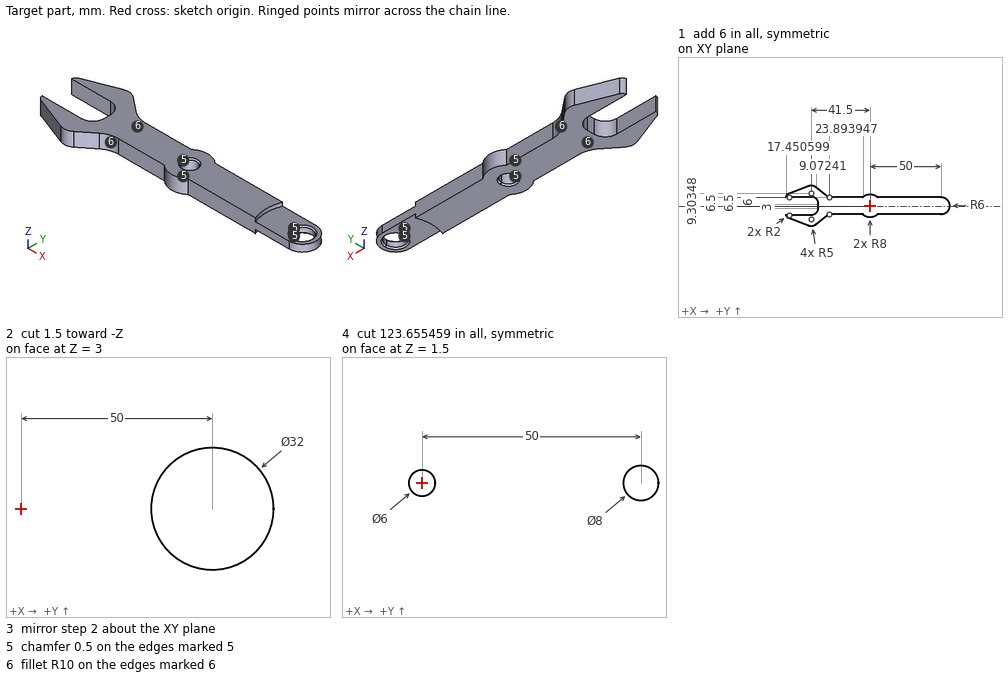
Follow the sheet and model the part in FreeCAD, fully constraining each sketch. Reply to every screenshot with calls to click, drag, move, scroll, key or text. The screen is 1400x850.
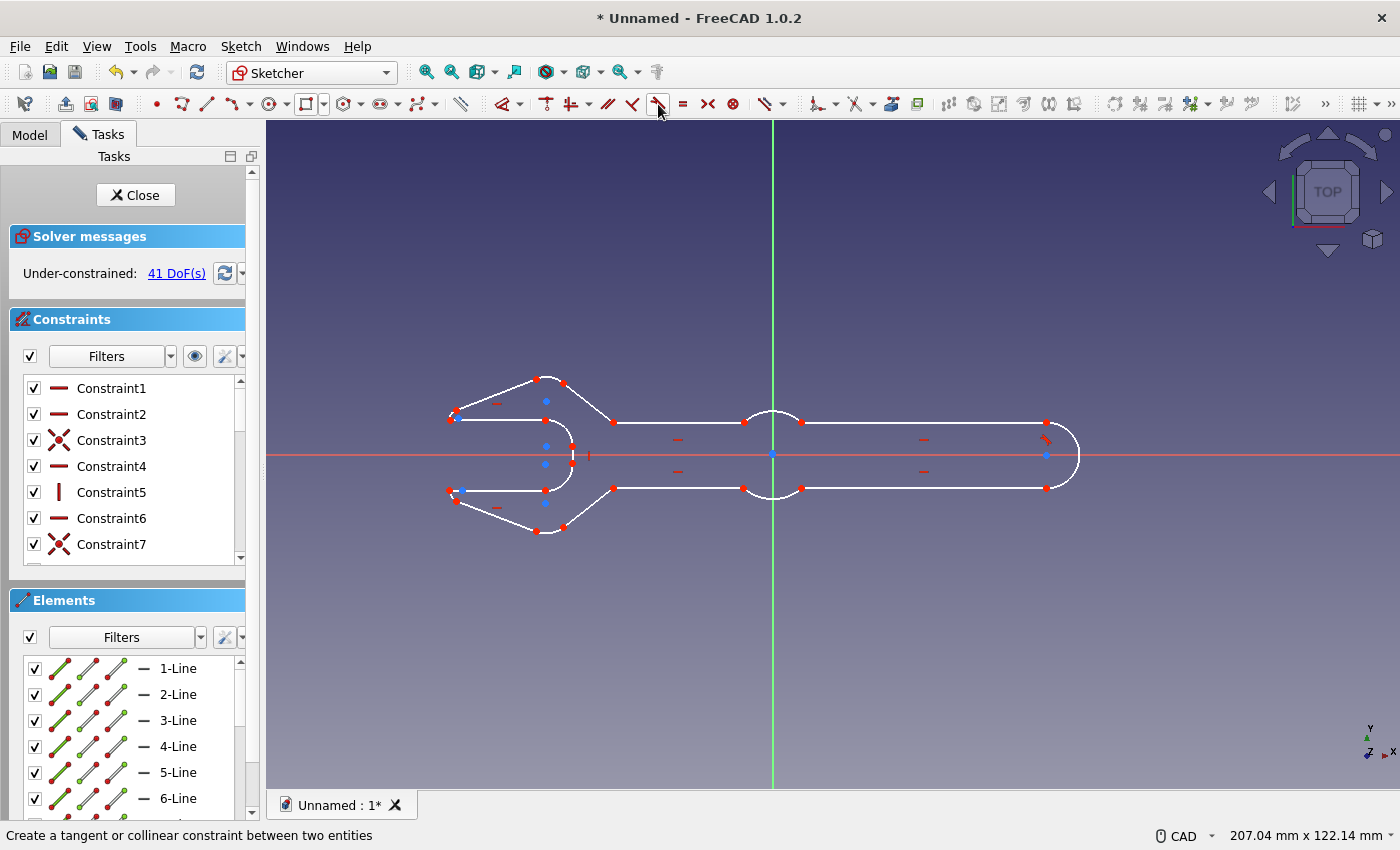
click(598, 411)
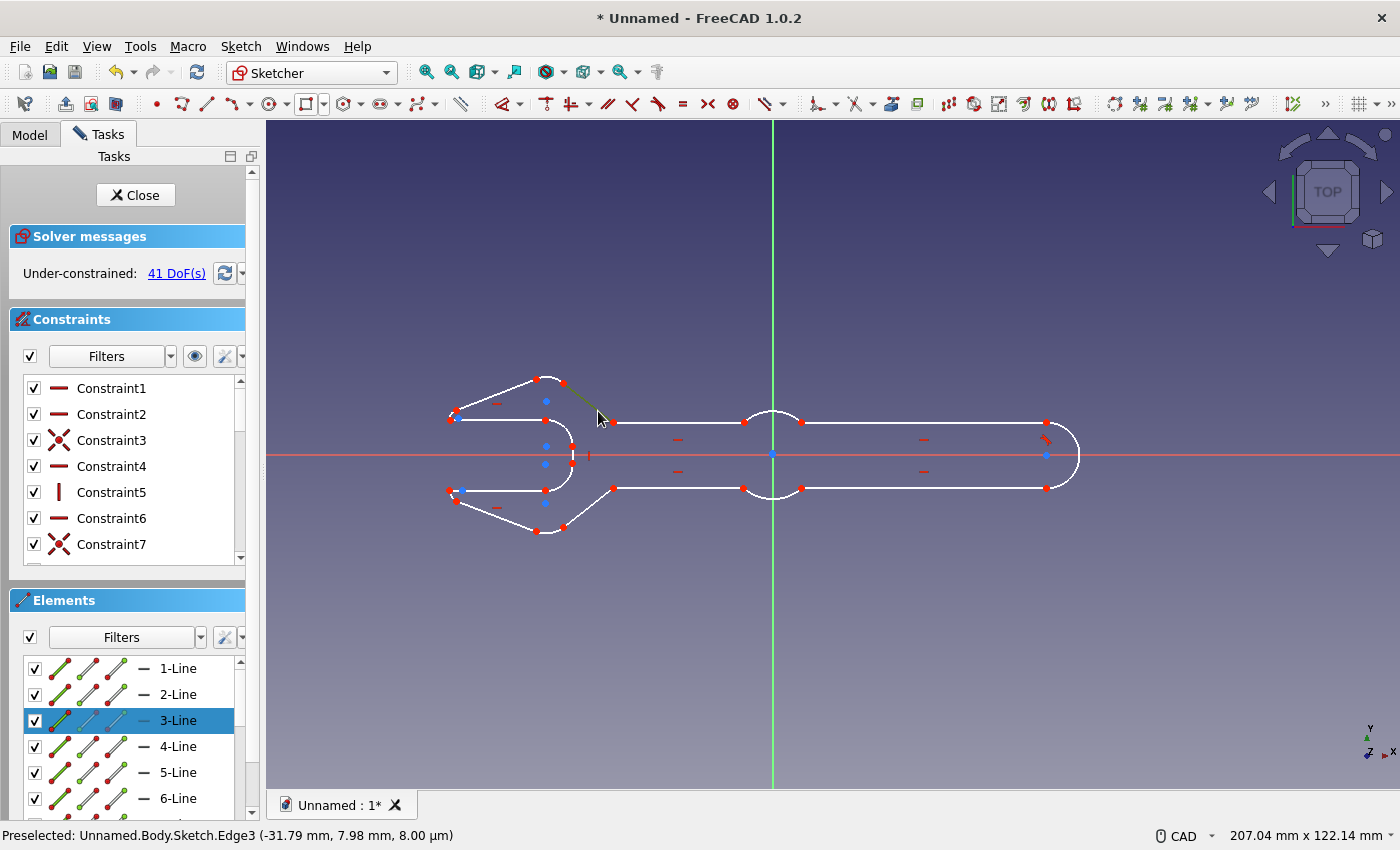
click(550, 377)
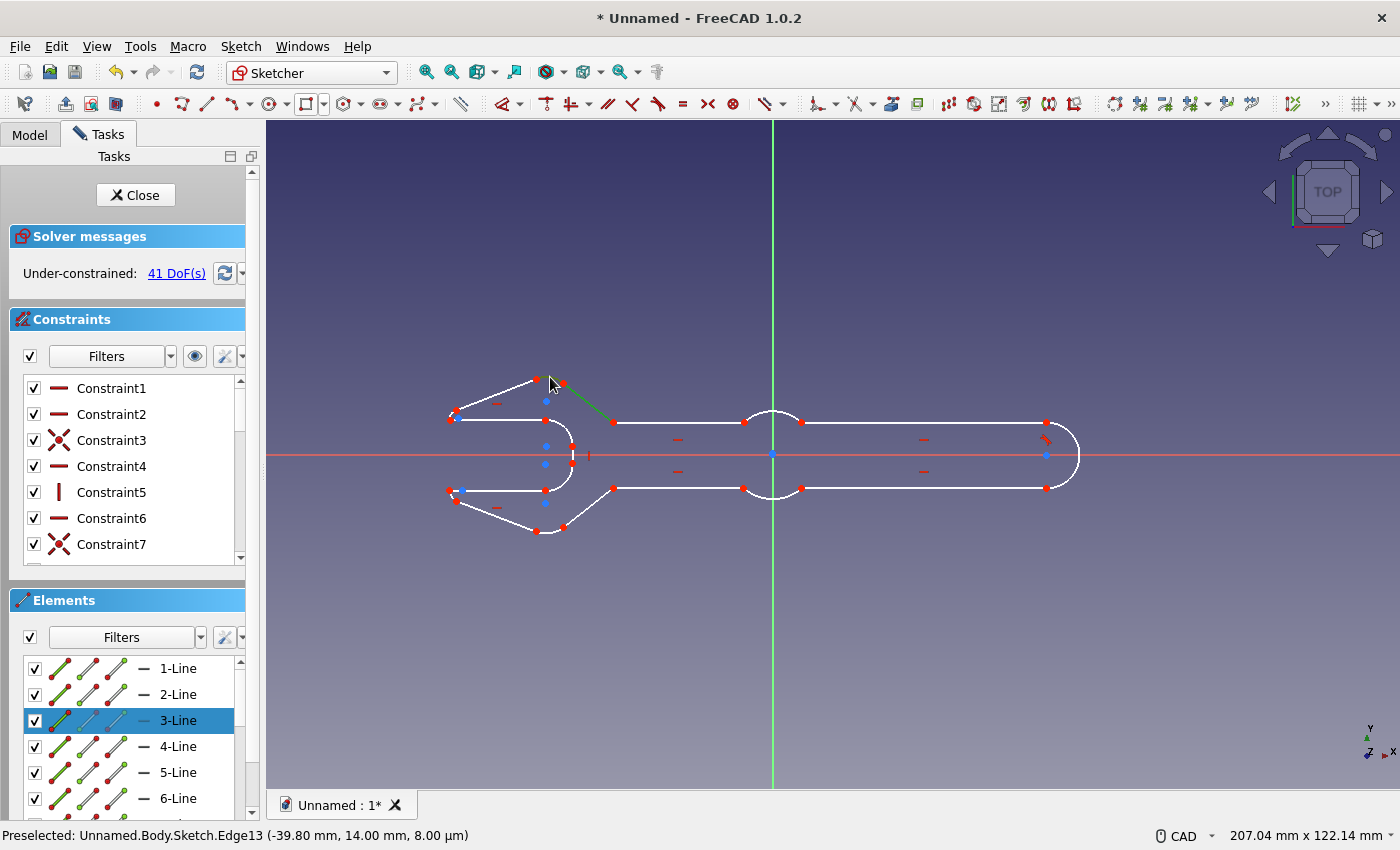
click(658, 104)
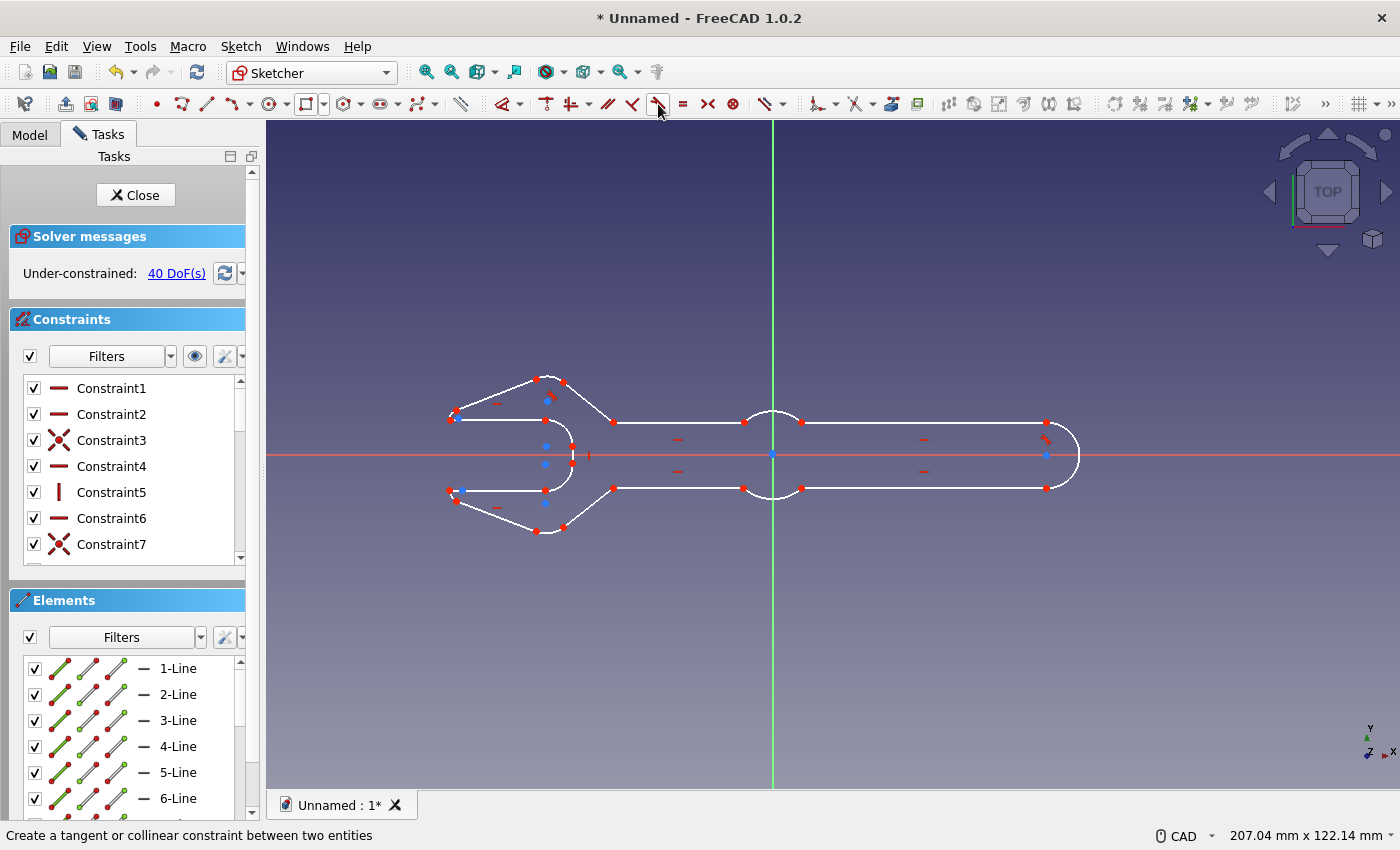
click(512, 389)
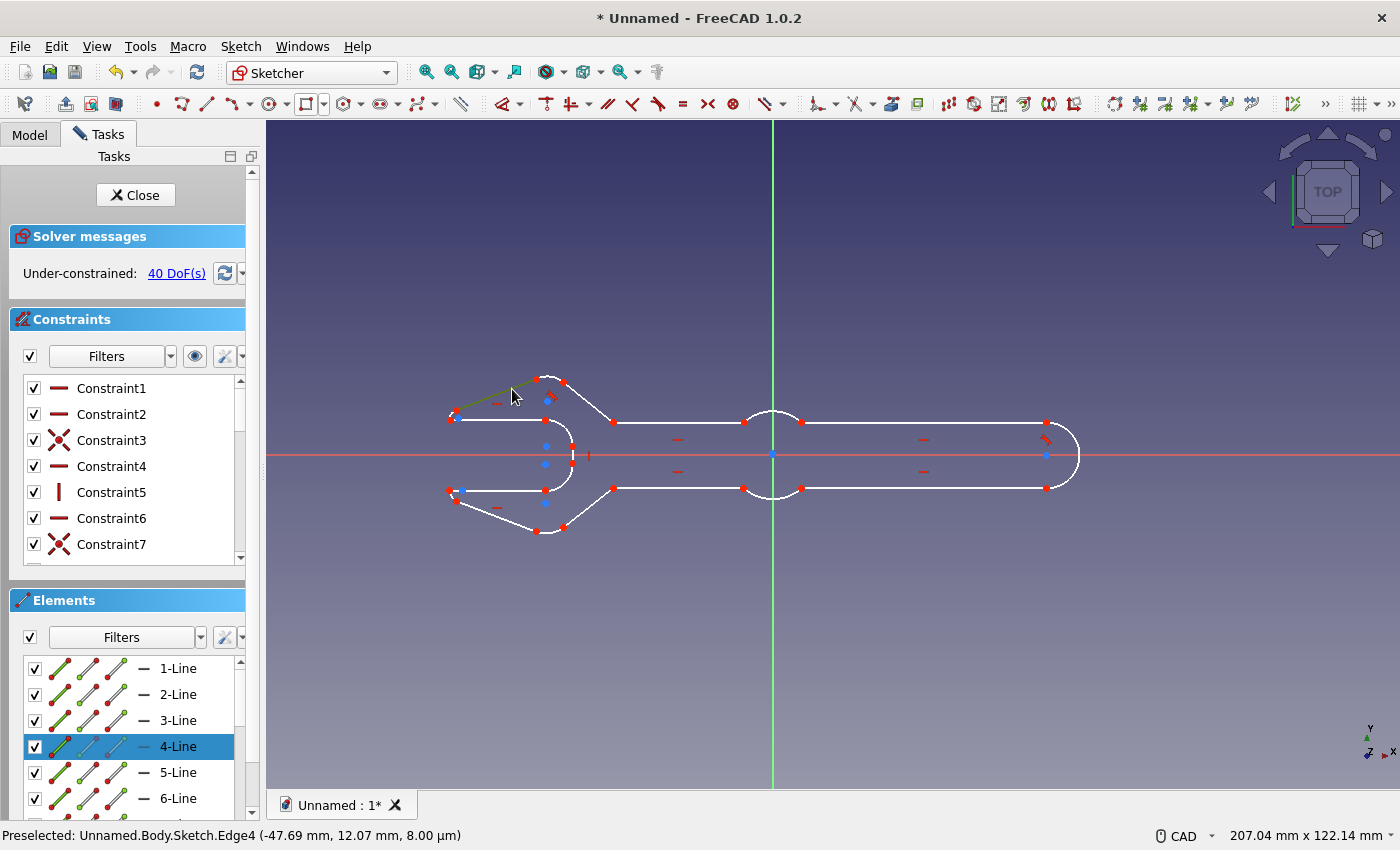
click(550, 377)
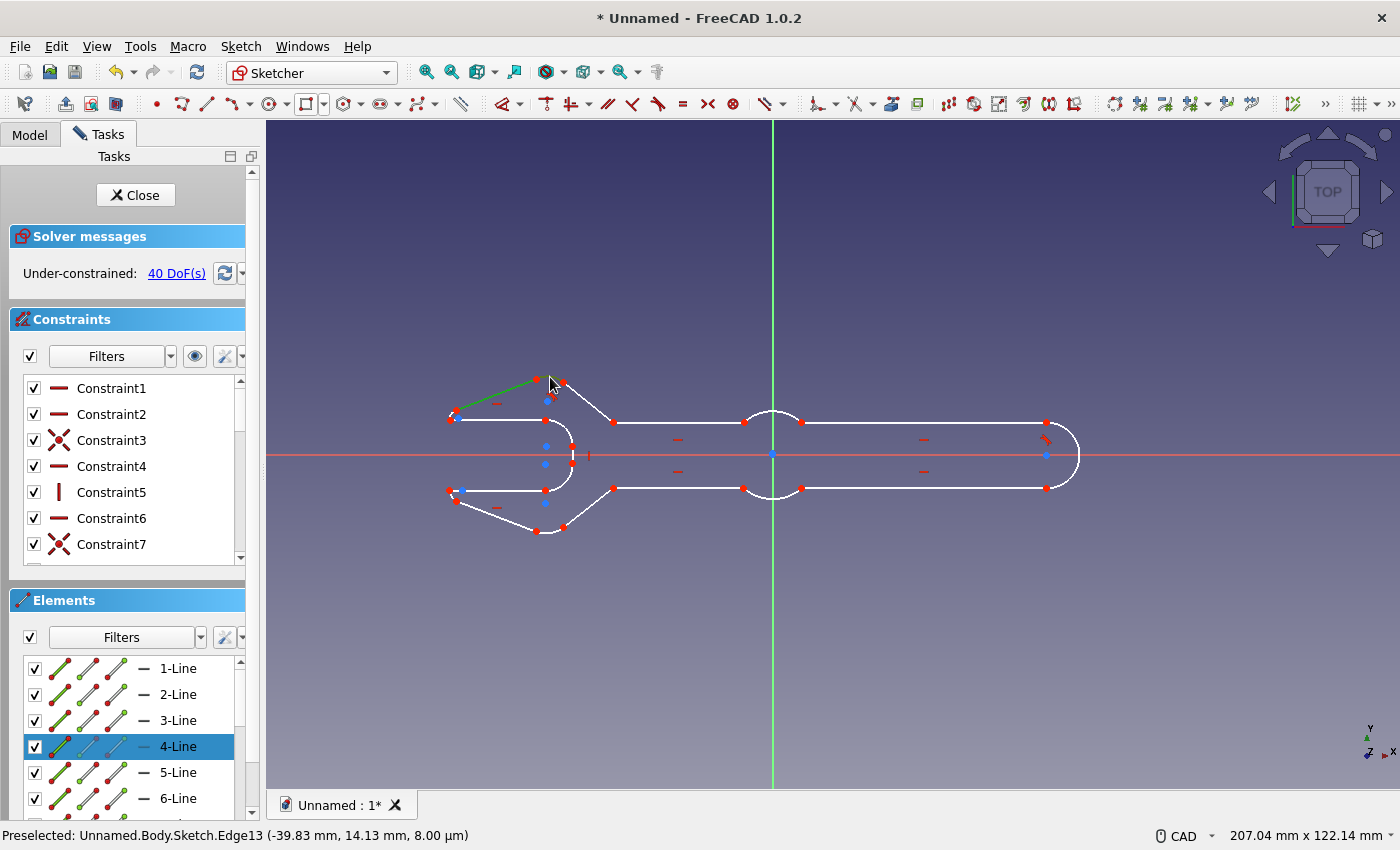
click(658, 104)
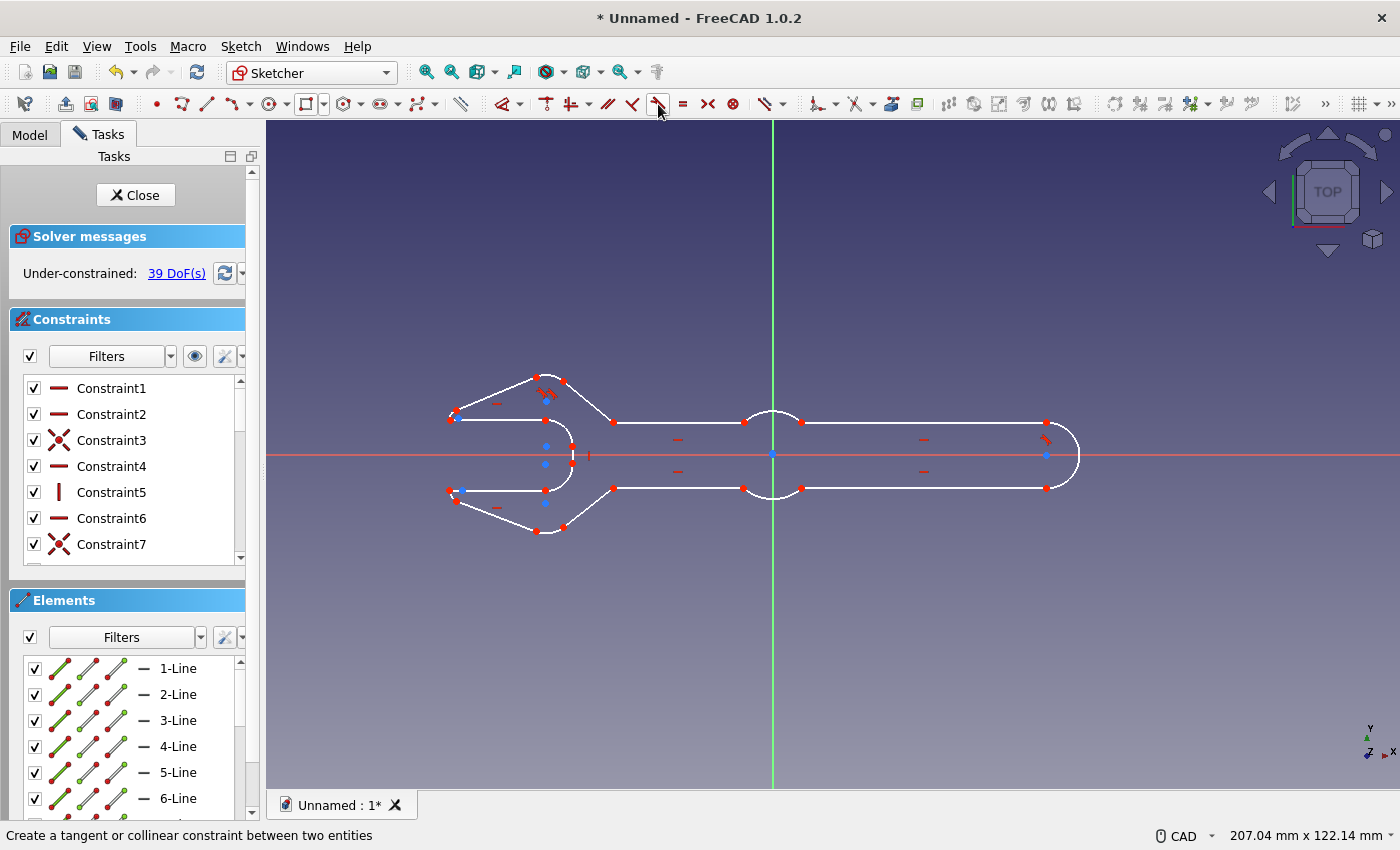
click(512, 387)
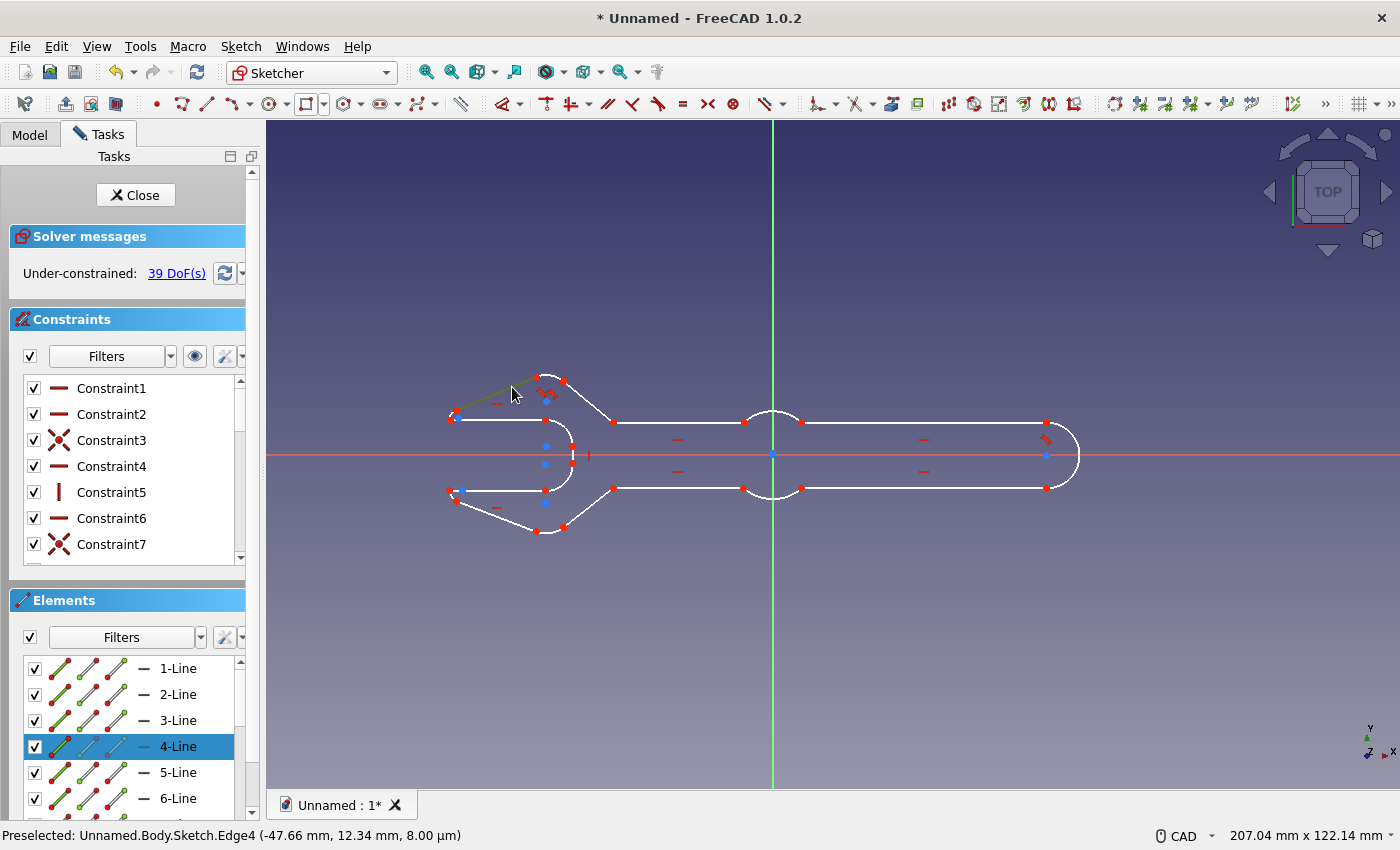
scroll(451, 414, up, 4)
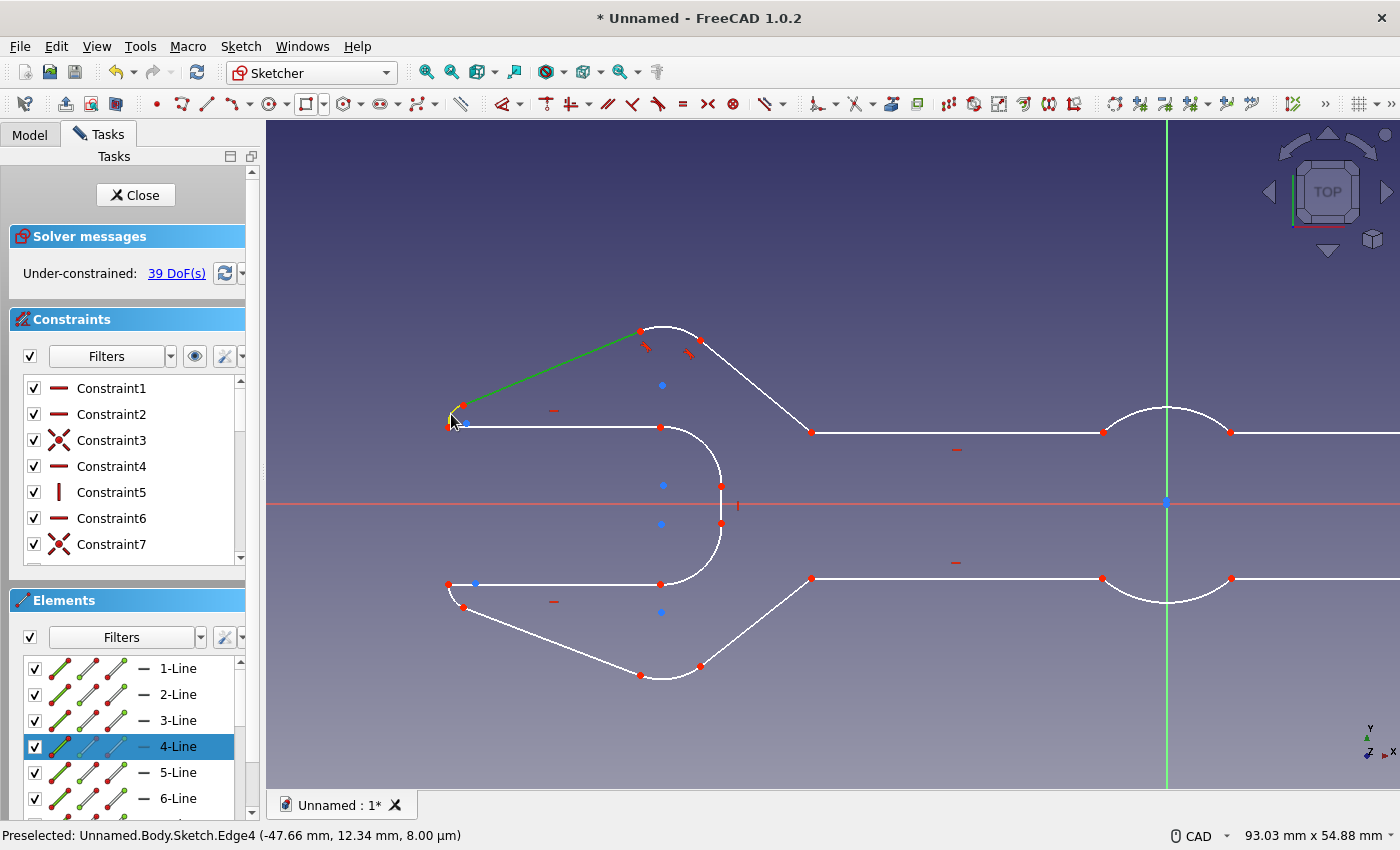
click(452, 413)